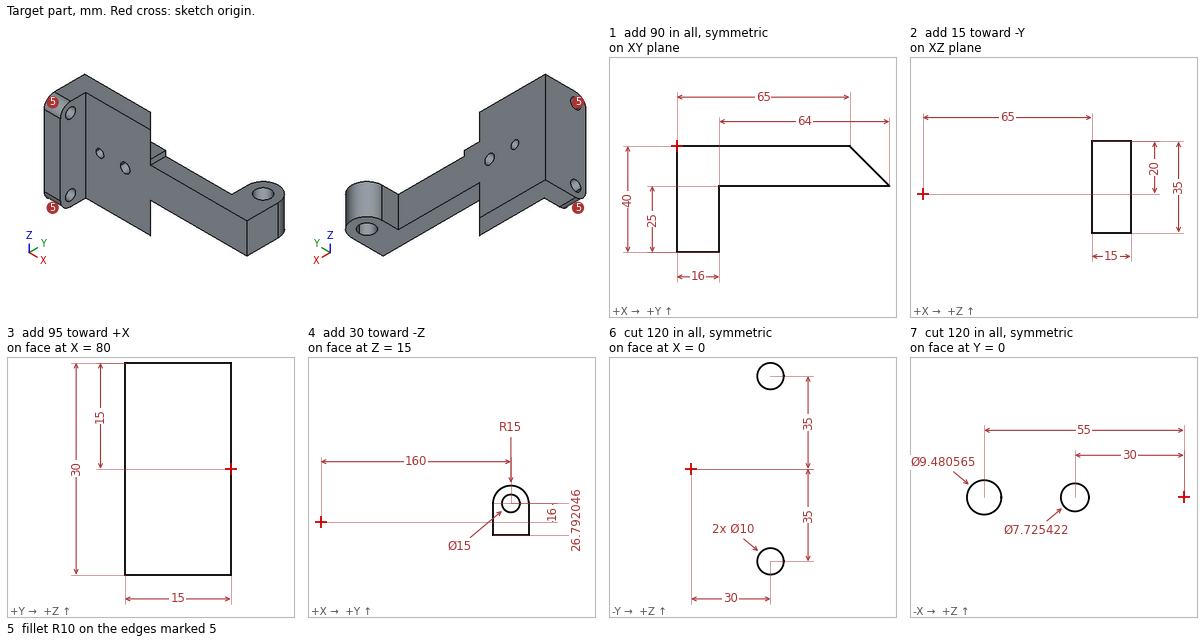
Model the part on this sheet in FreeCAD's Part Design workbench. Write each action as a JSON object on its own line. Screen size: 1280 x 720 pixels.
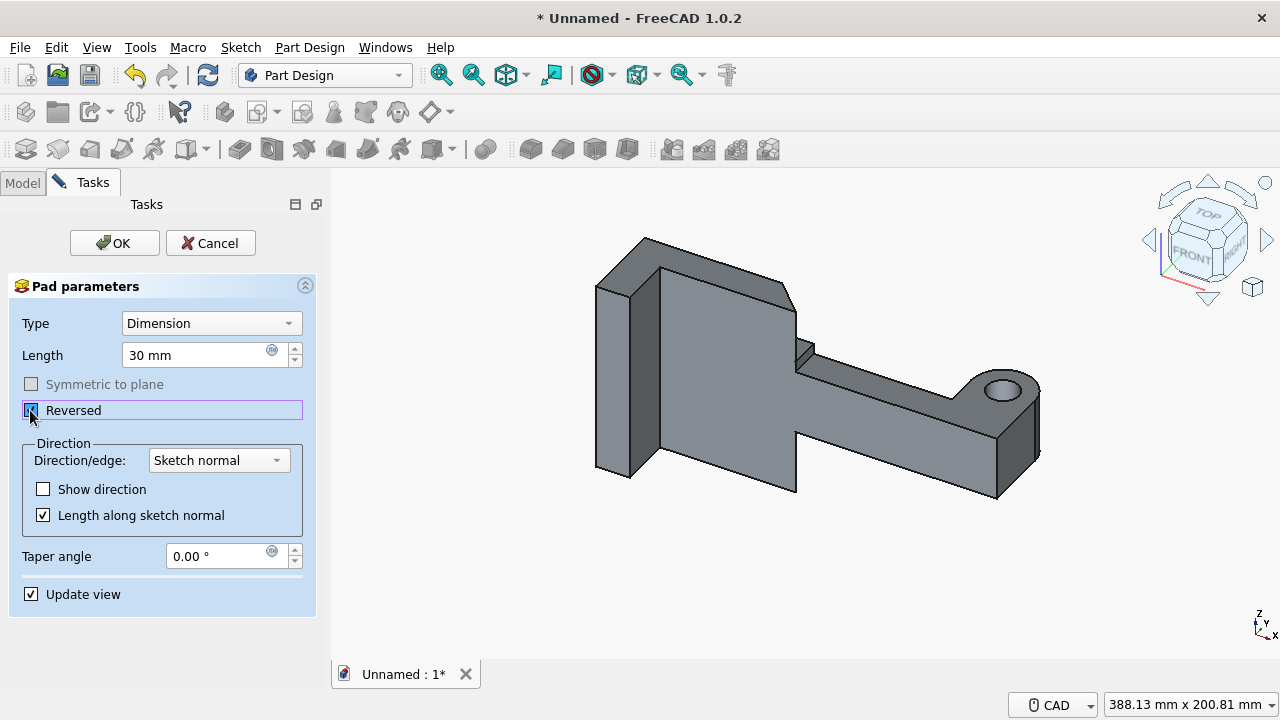
{"action": "left_click", "coordinate": [115, 243]}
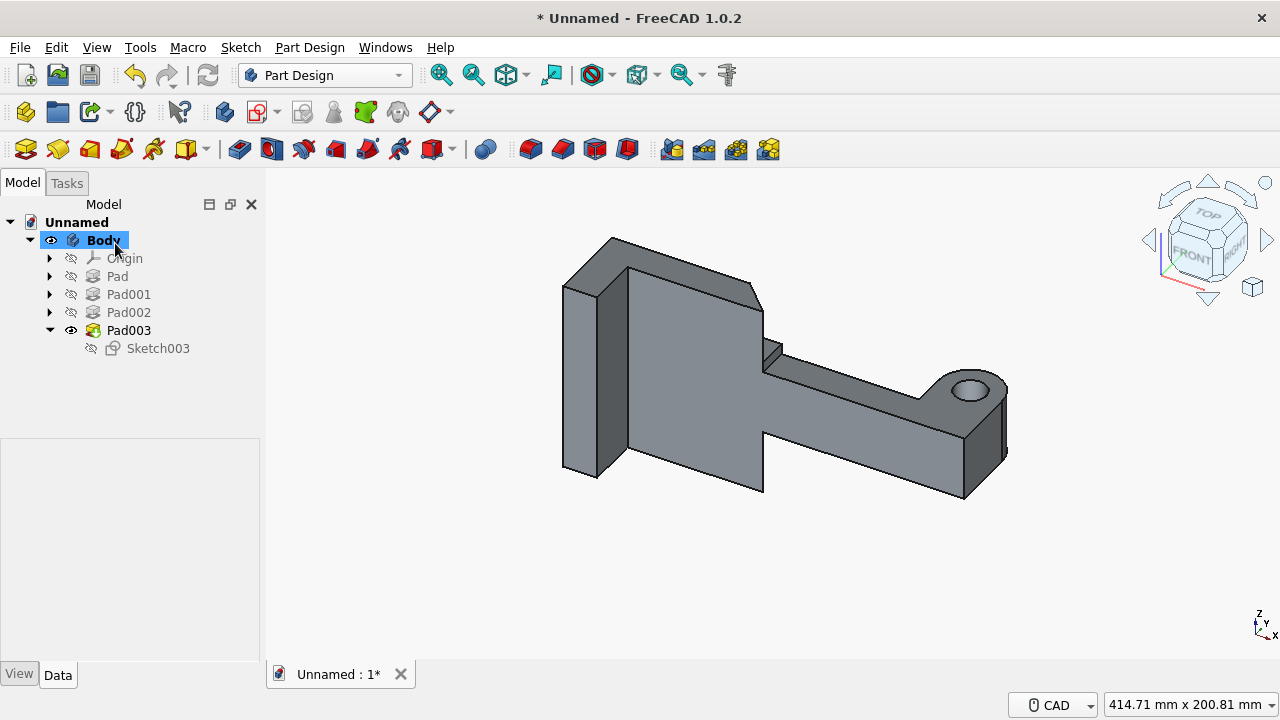
{"action": "left_click", "coordinate": [580, 291]}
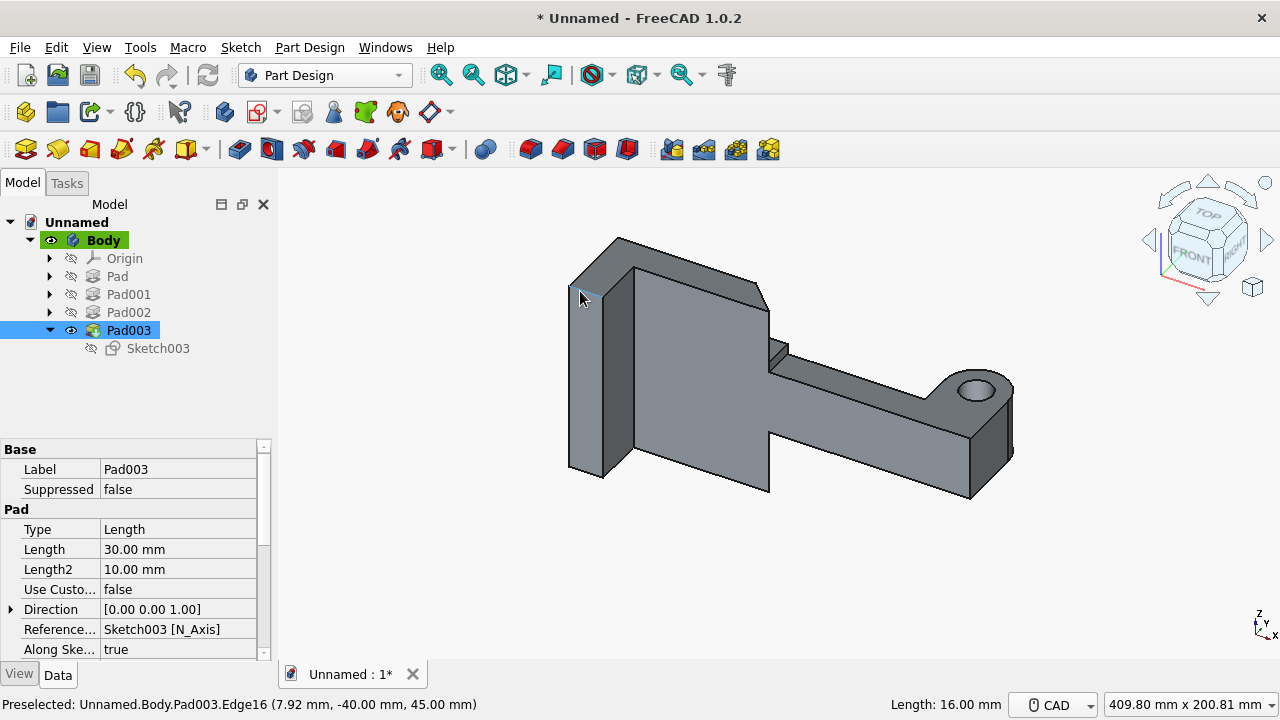
{"action": "key", "text": "0"}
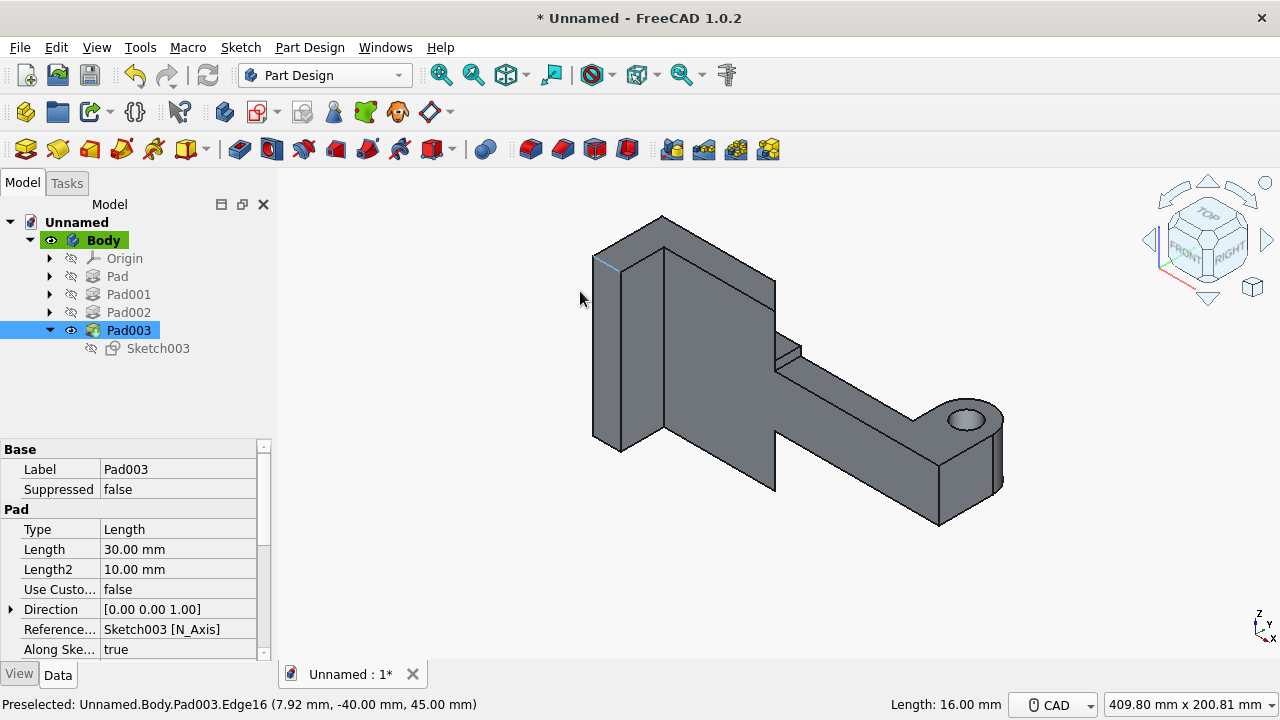
{"action": "key", "text": "2"}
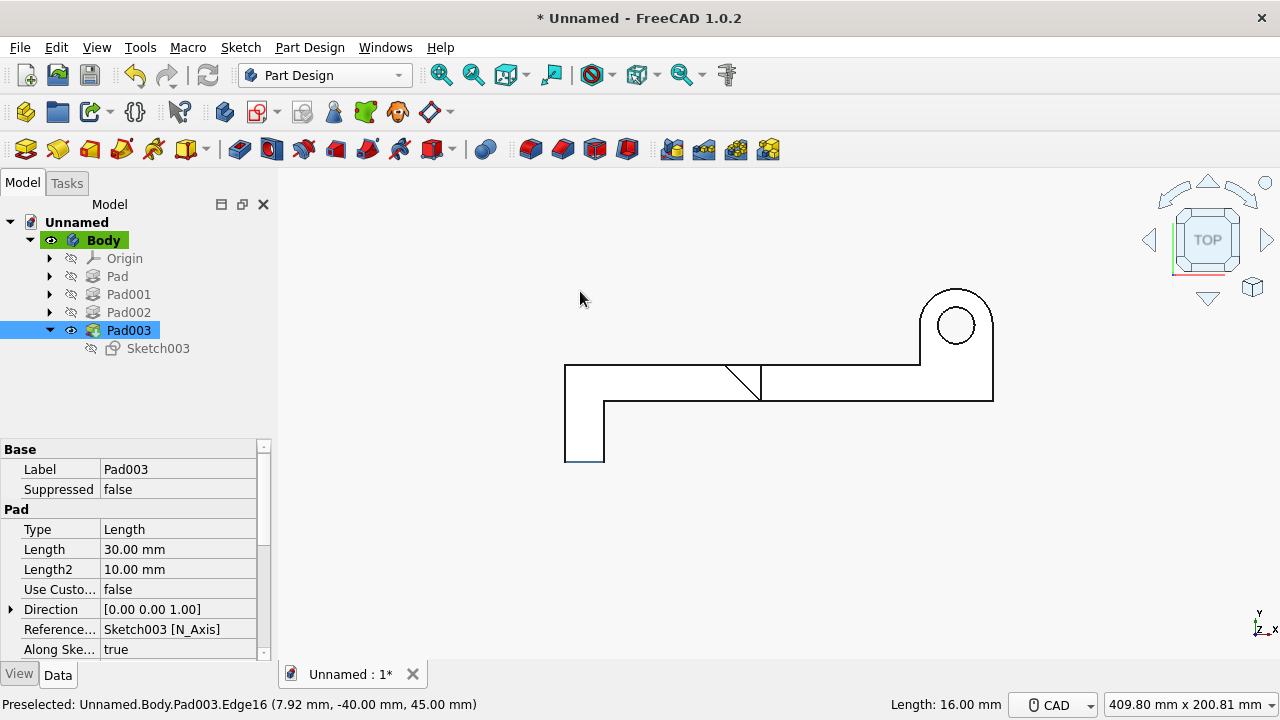
{"action": "left_click", "coordinate": [442, 76]}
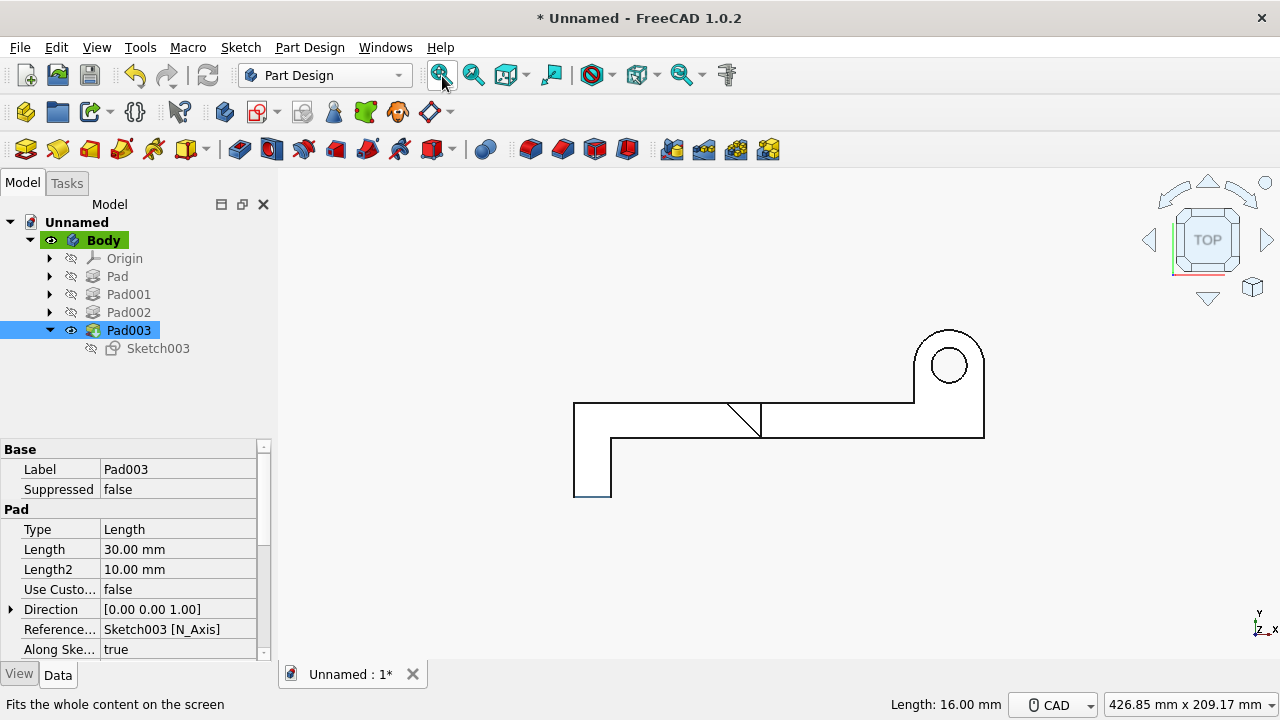
{"action": "key", "text": "1"}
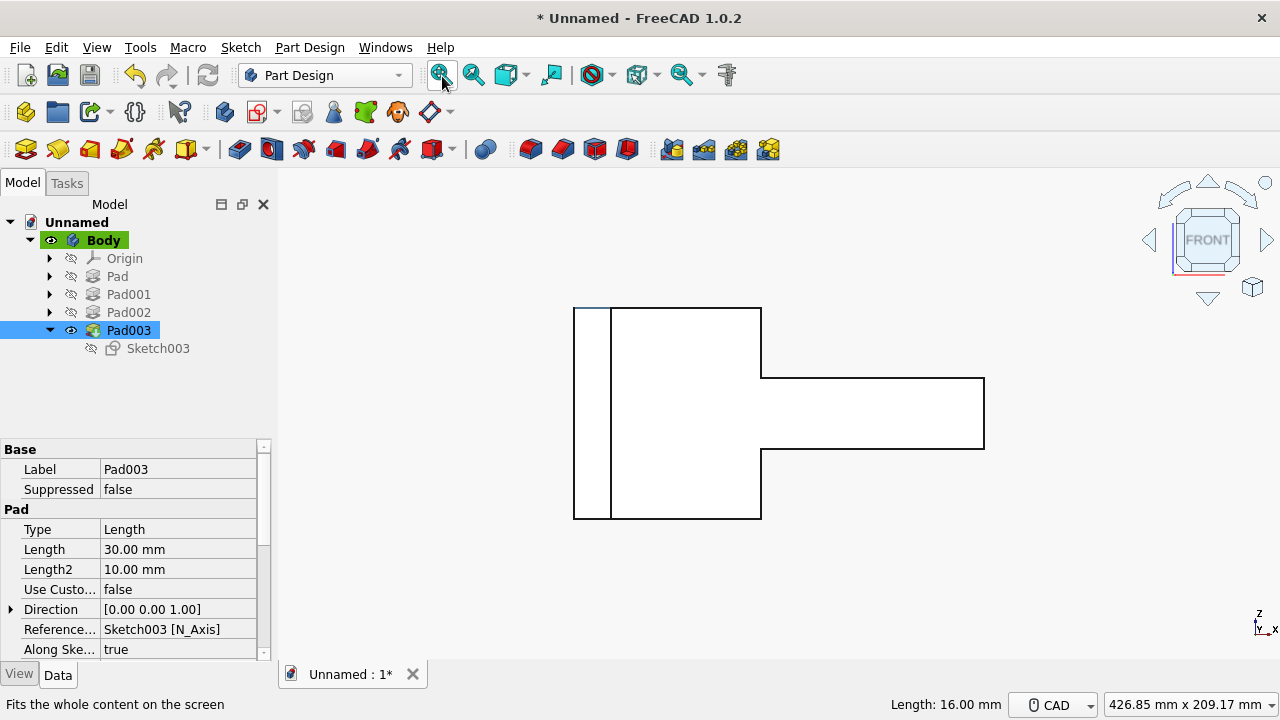
{"action": "left_click", "coordinate": [442, 76]}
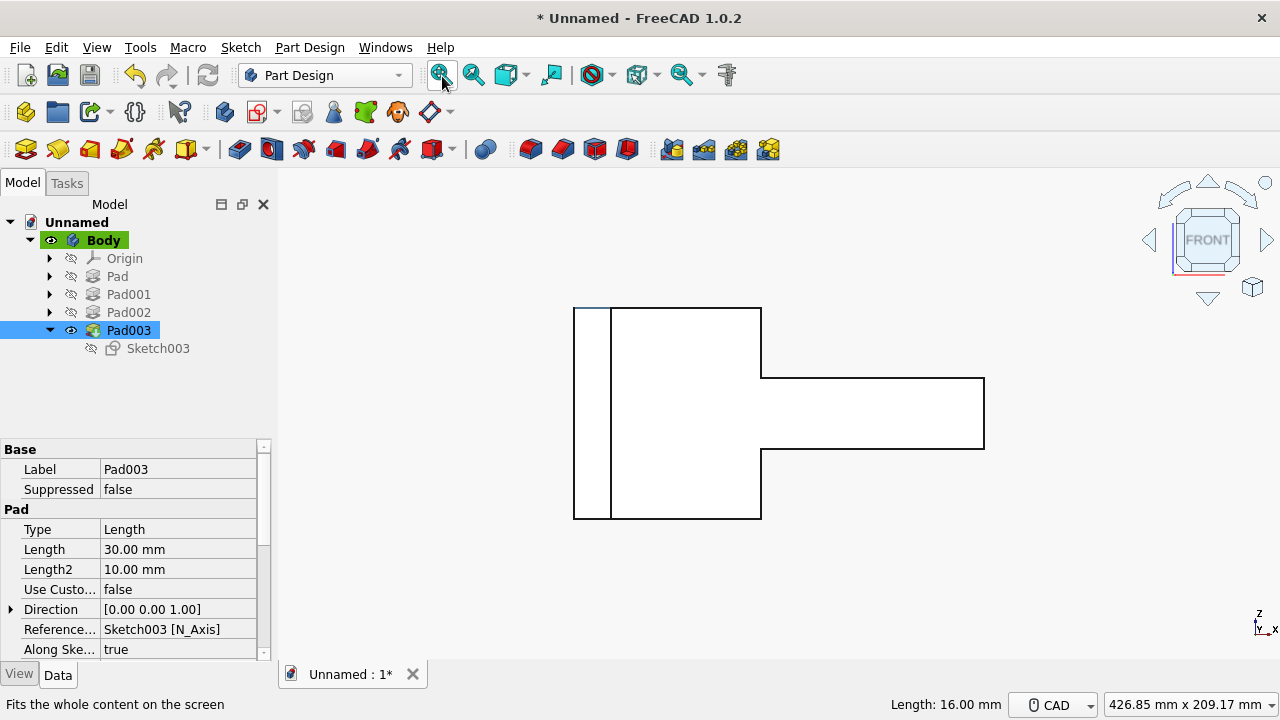
{"action": "left_click", "coordinate": [592, 518], "text": "ctrl"}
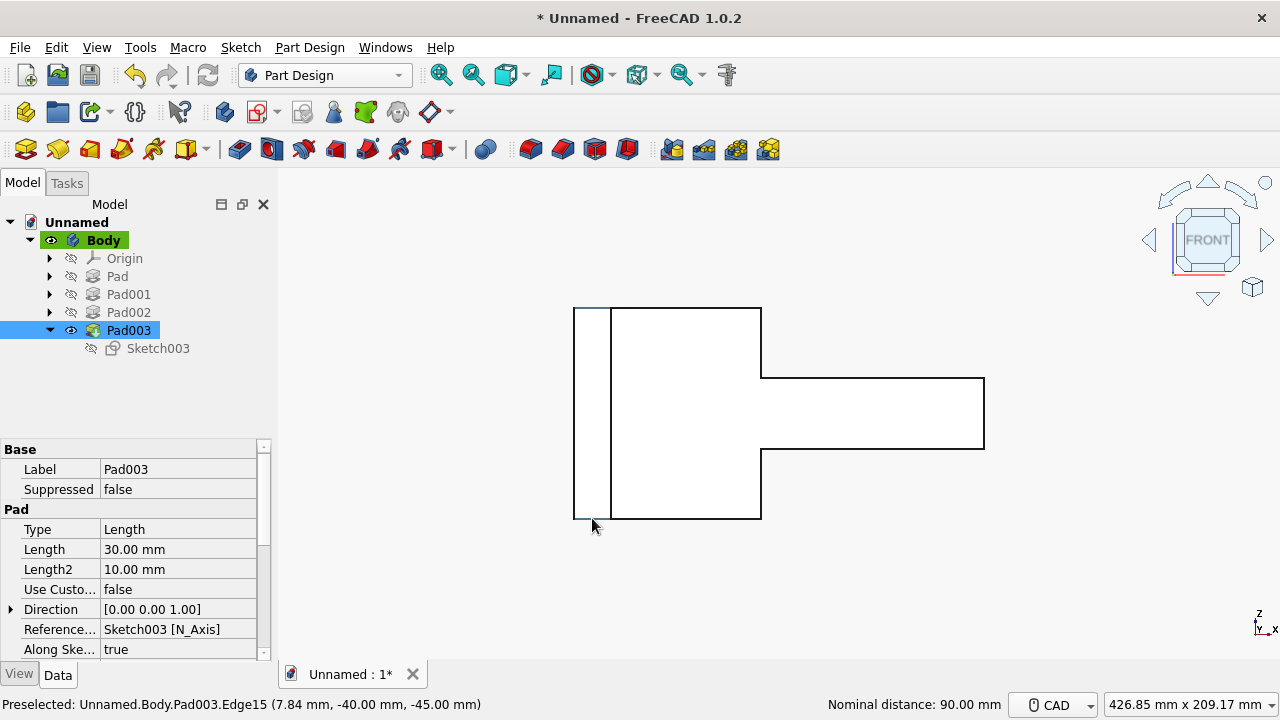
{"action": "left_click", "coordinate": [532, 150]}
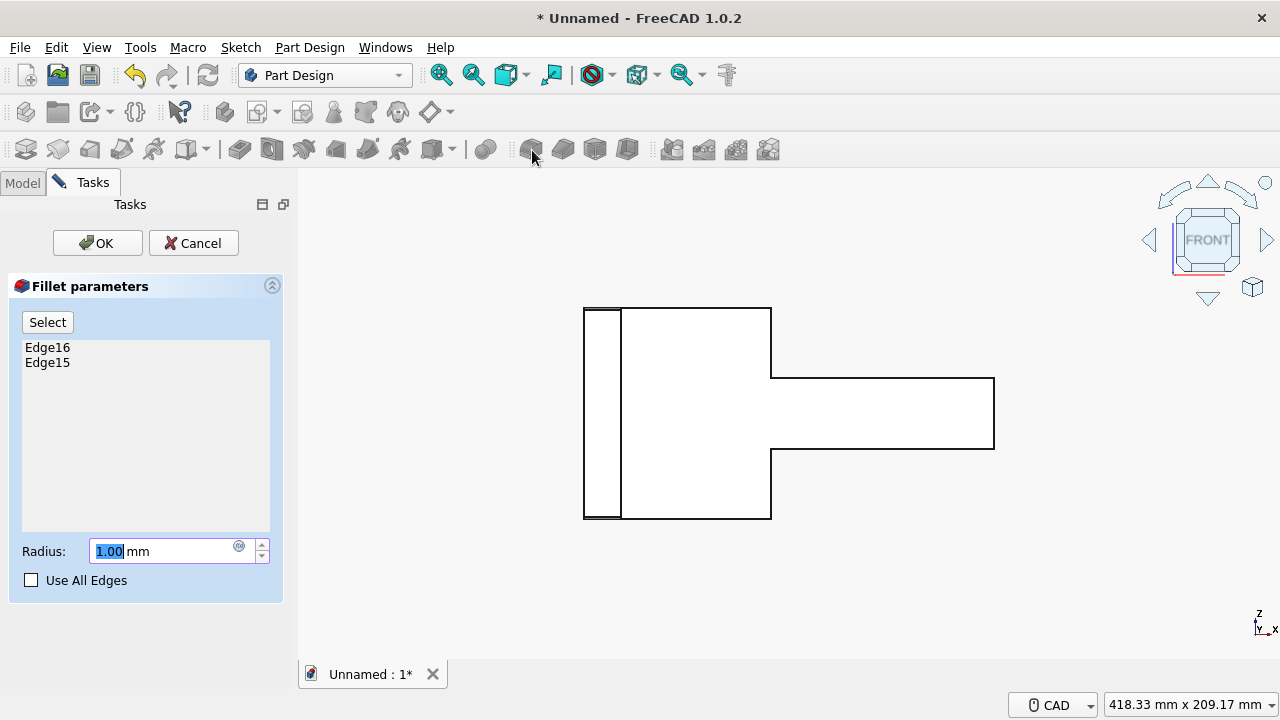
{"action": "type", "text": "10"}
{"action": "key", "text": "Tab"}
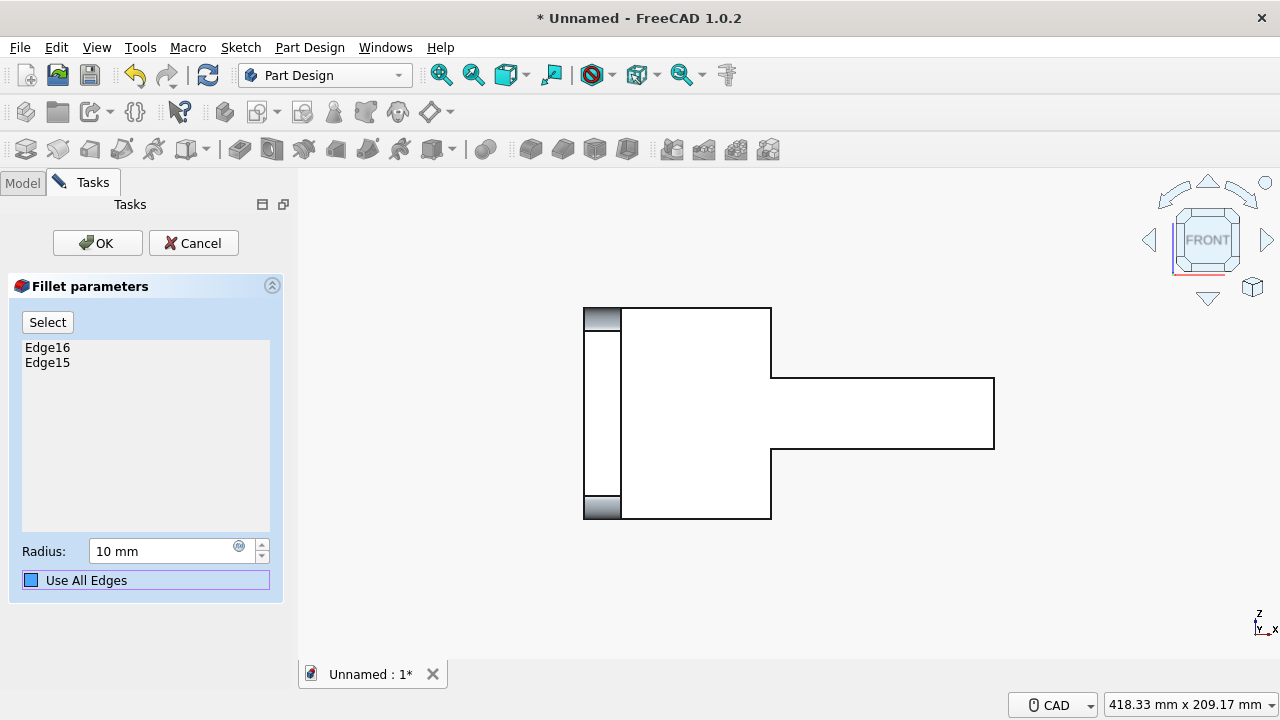
{"action": "left_click", "coordinate": [98, 243]}